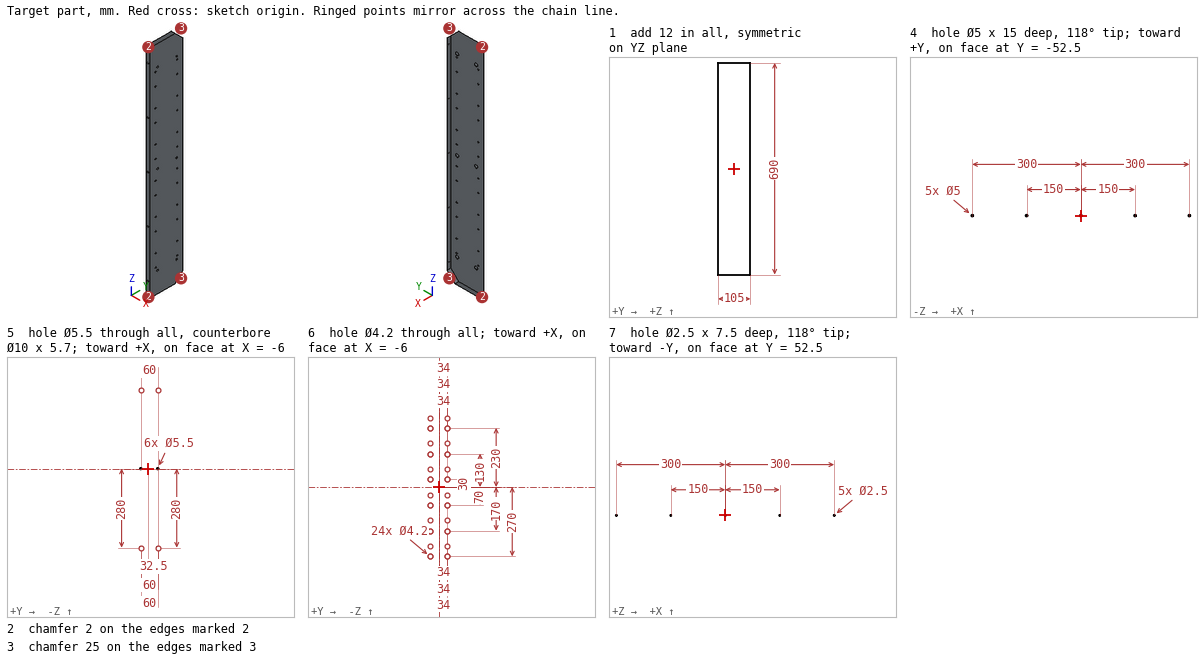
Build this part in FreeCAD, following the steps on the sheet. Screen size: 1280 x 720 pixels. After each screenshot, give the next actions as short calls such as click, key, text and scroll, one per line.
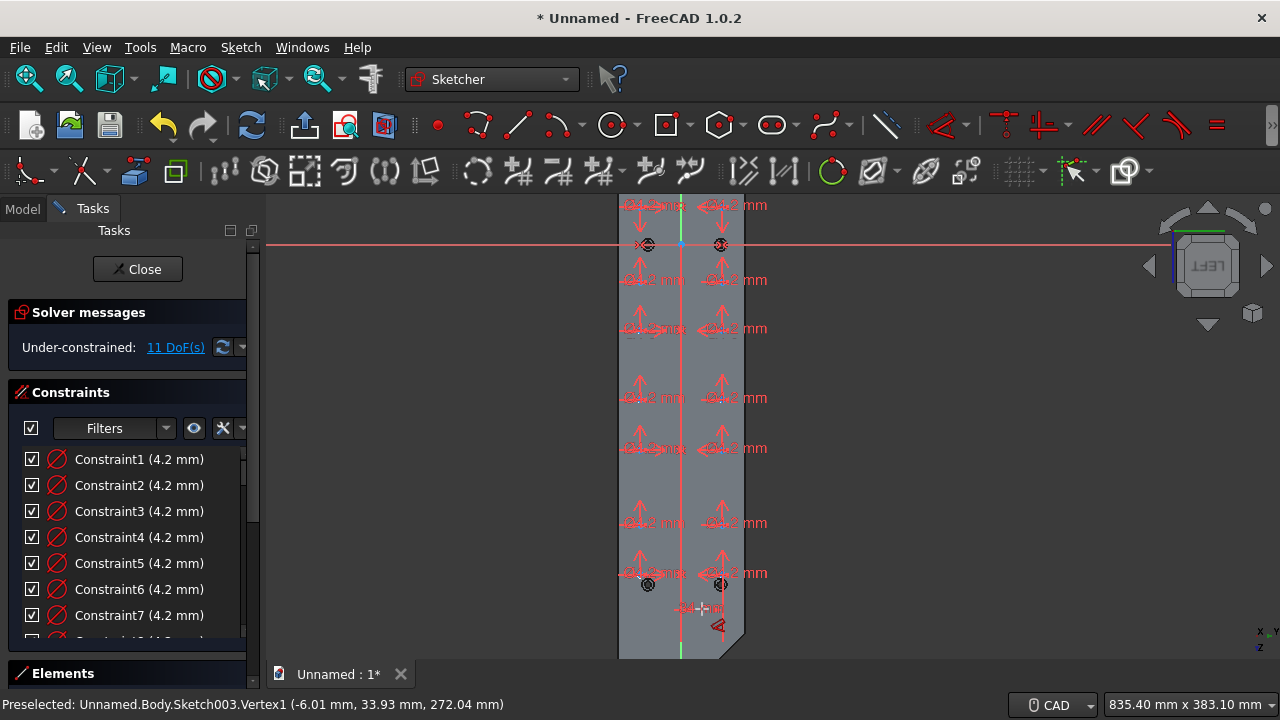
click(722, 450)
click(702, 484)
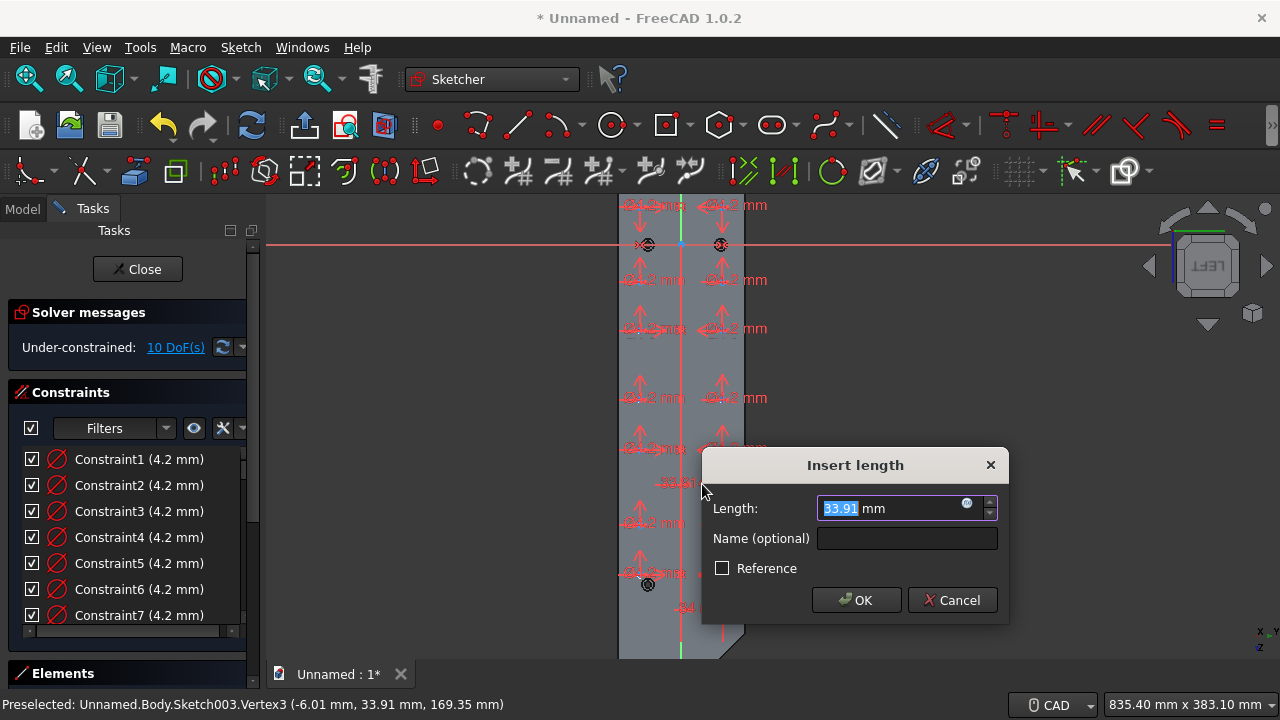
text(34)
key(Return)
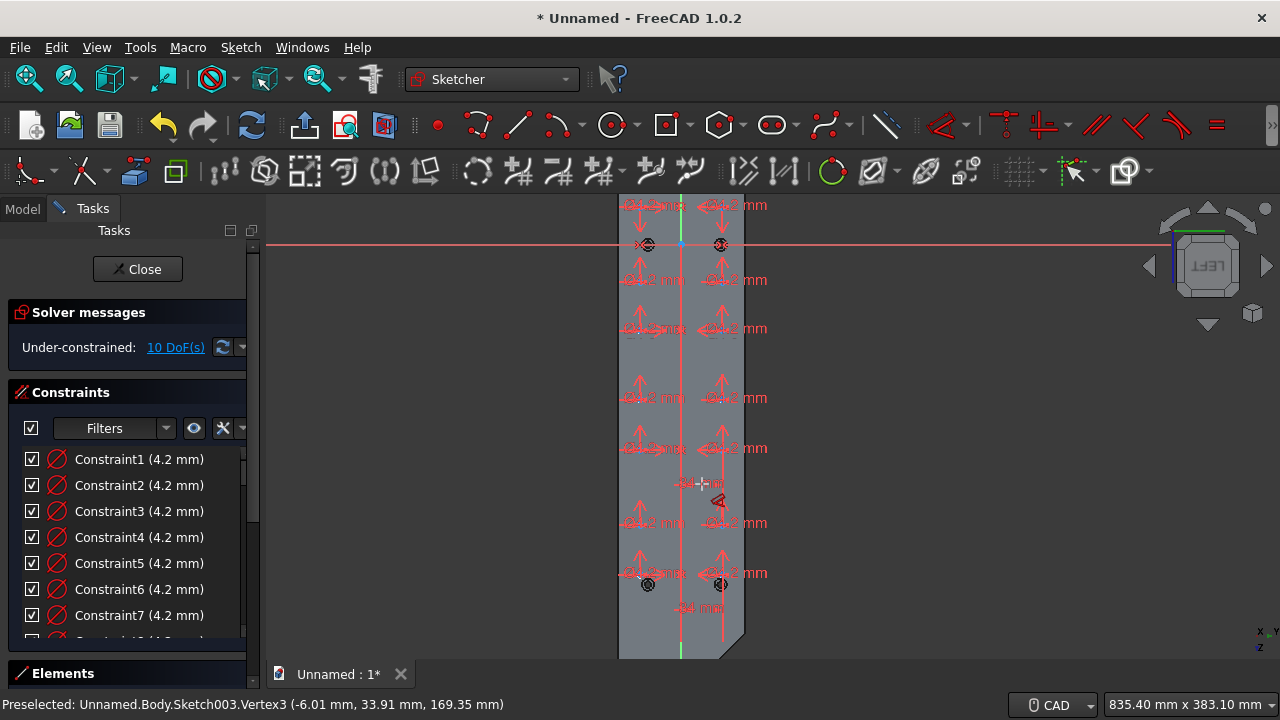
click(722, 331)
click(702, 365)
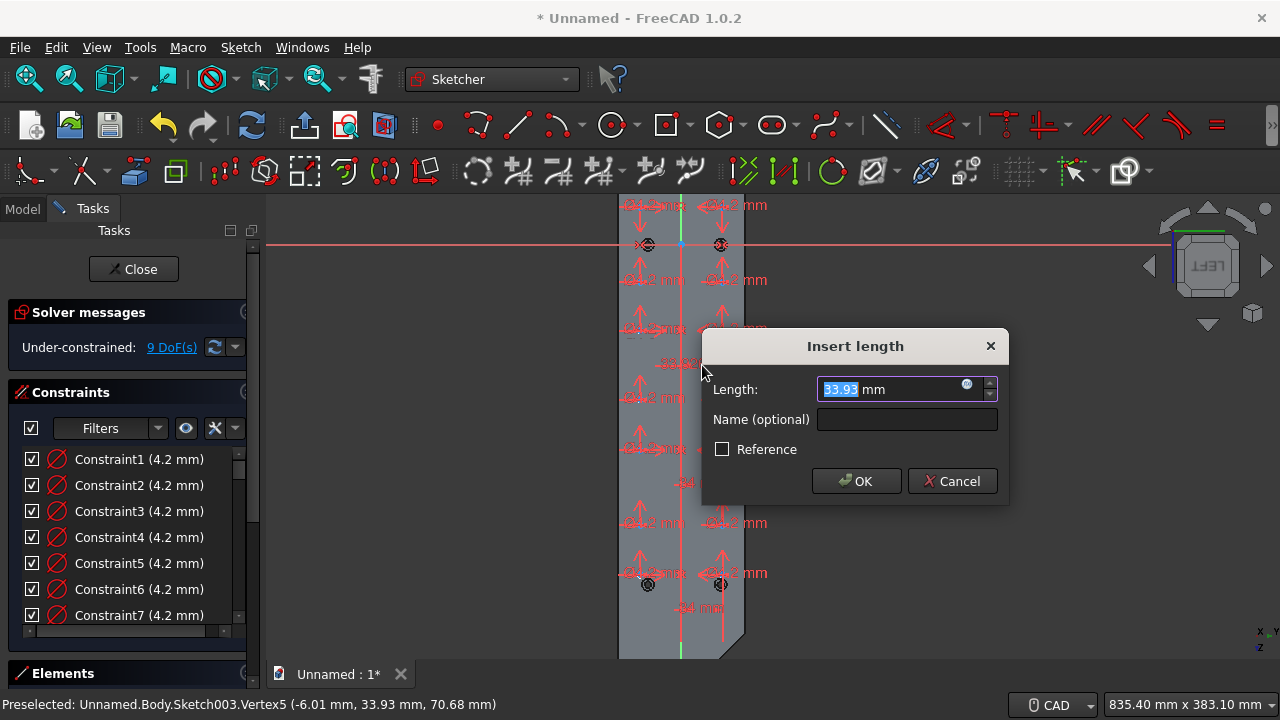
text(34)
key(Return)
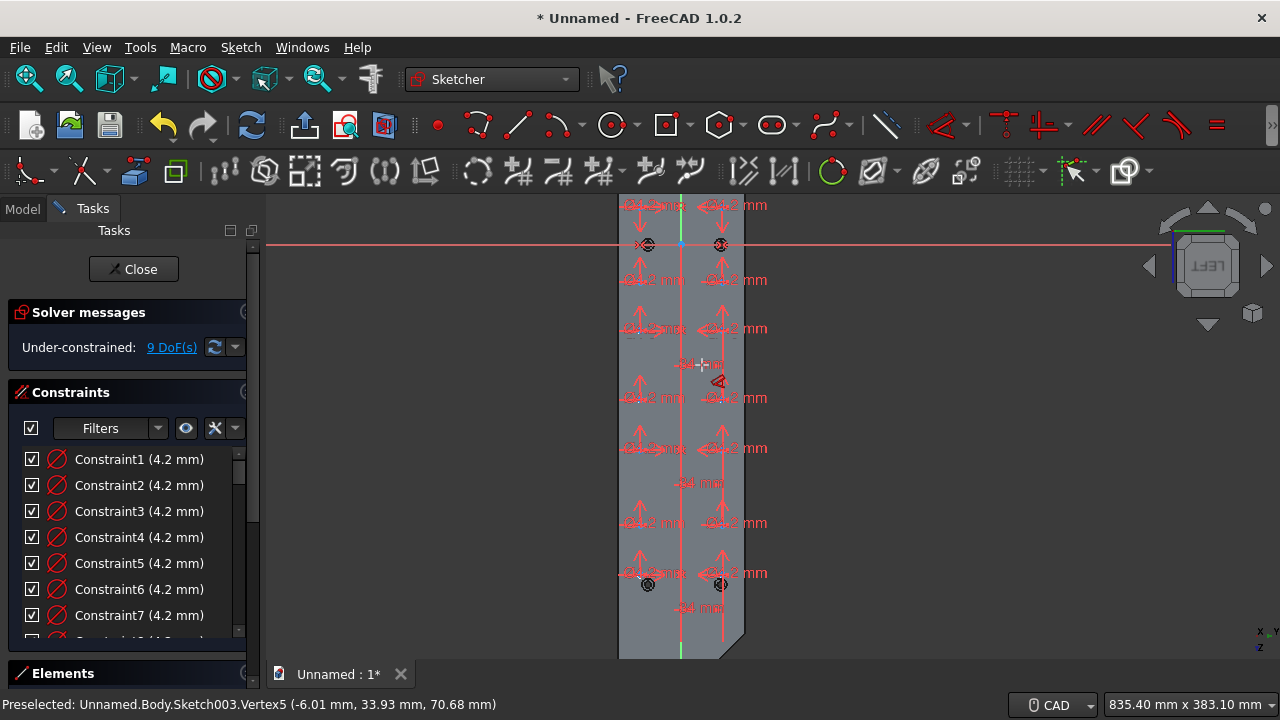
click(723, 331)
click(757, 288)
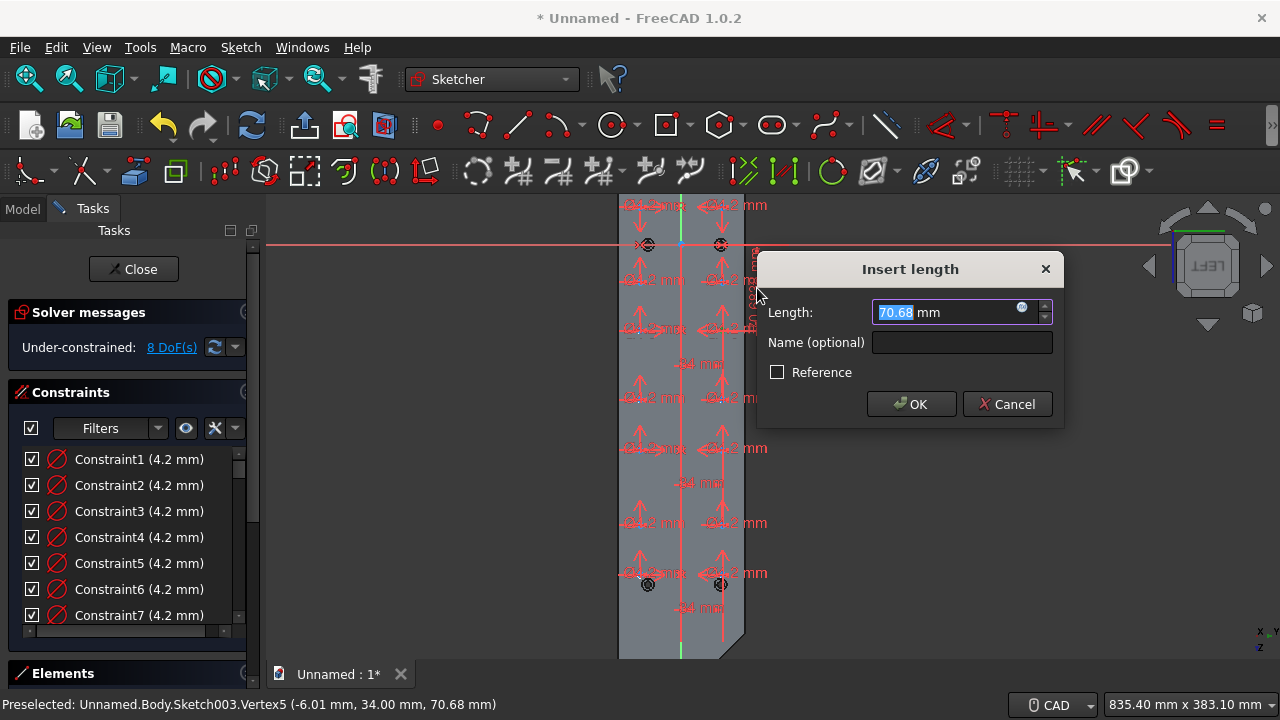
text(70)
key(Return)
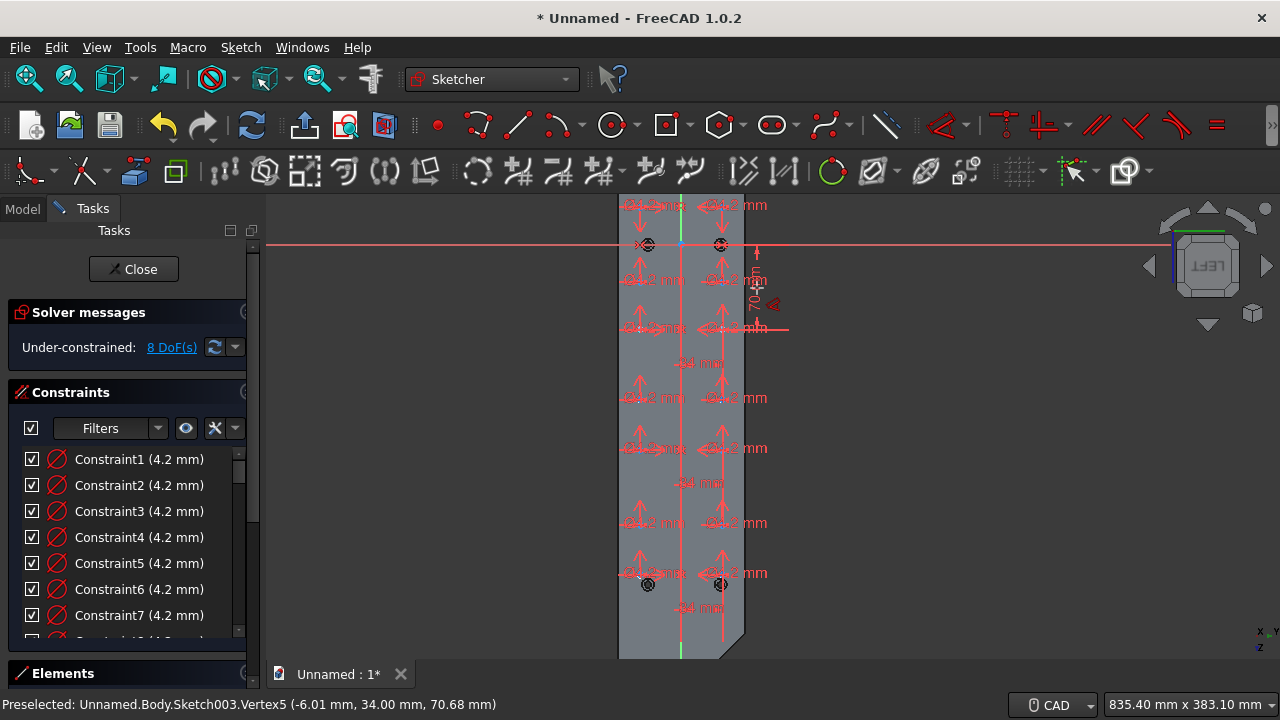
scroll(723, 575, down, 4)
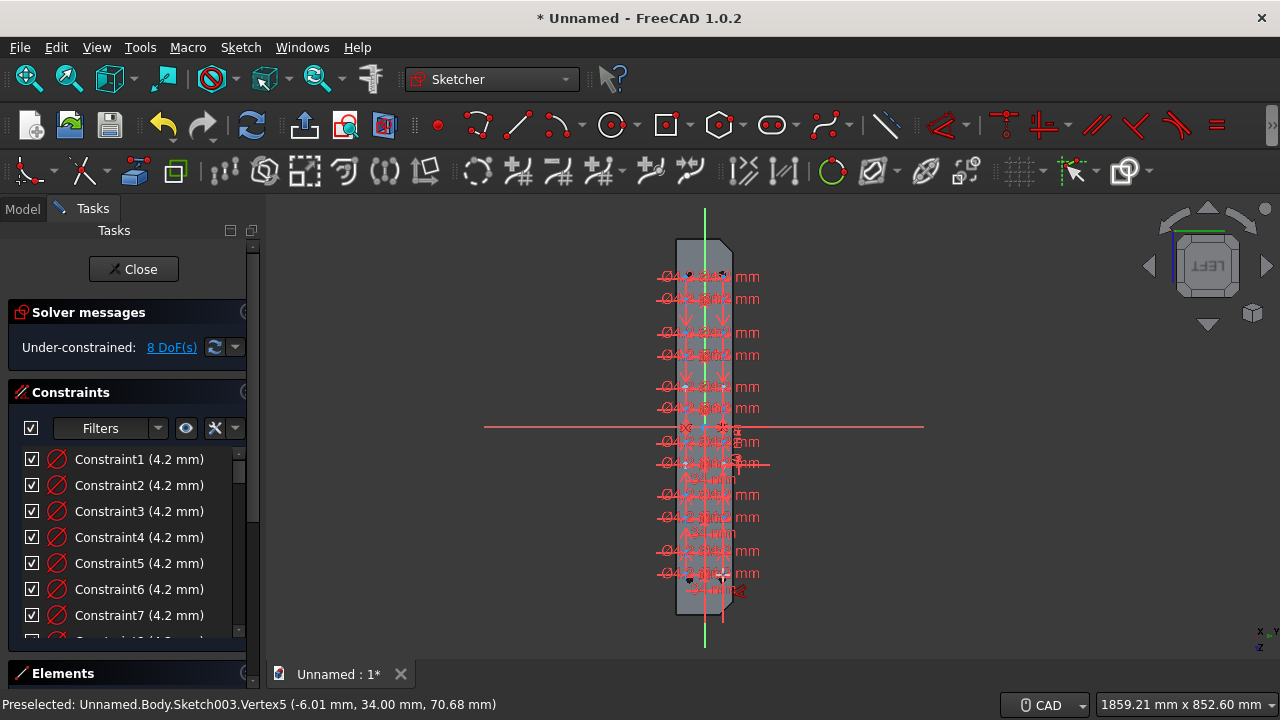
scroll(723, 410, up, 4)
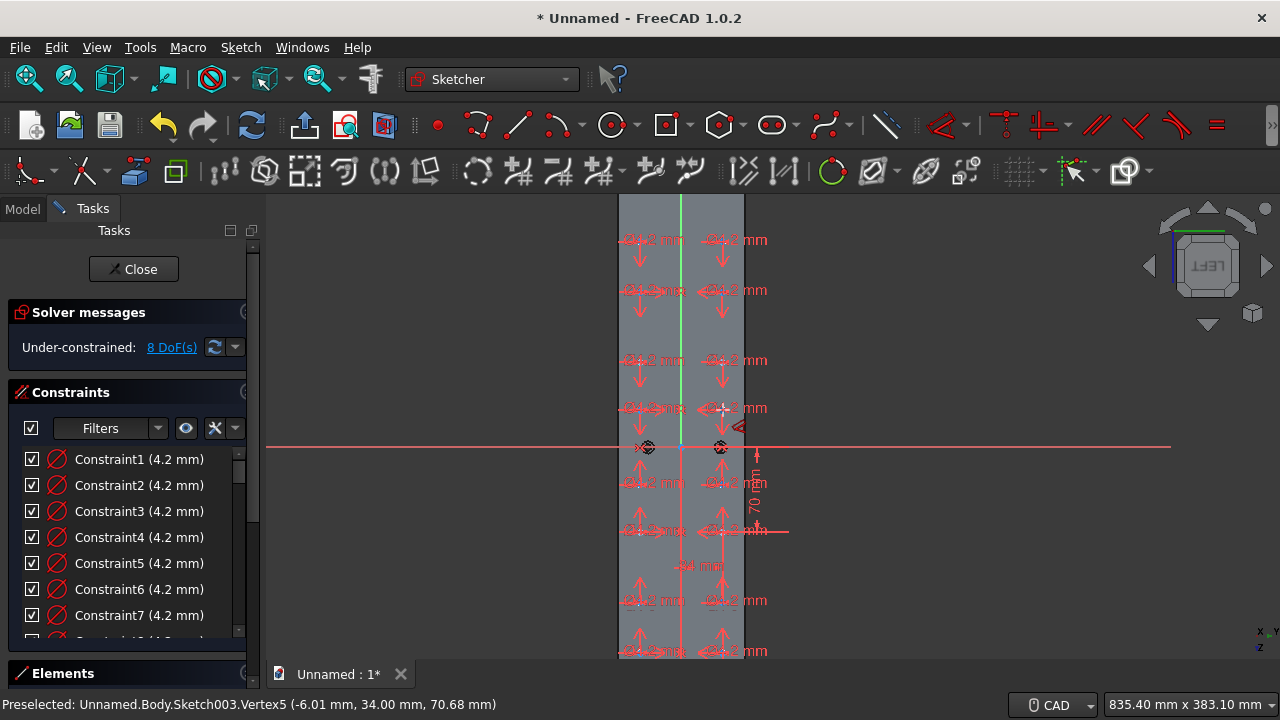
click(722, 410)
click(702, 376)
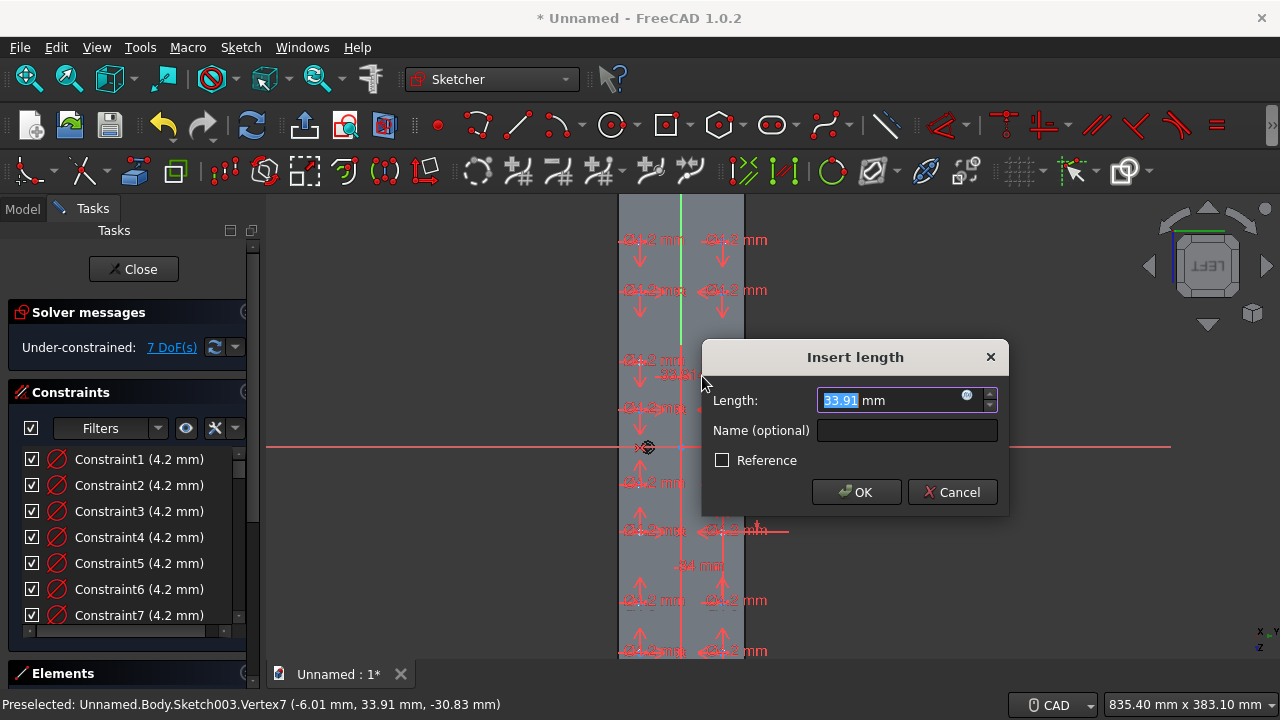
text(34)
key(Return)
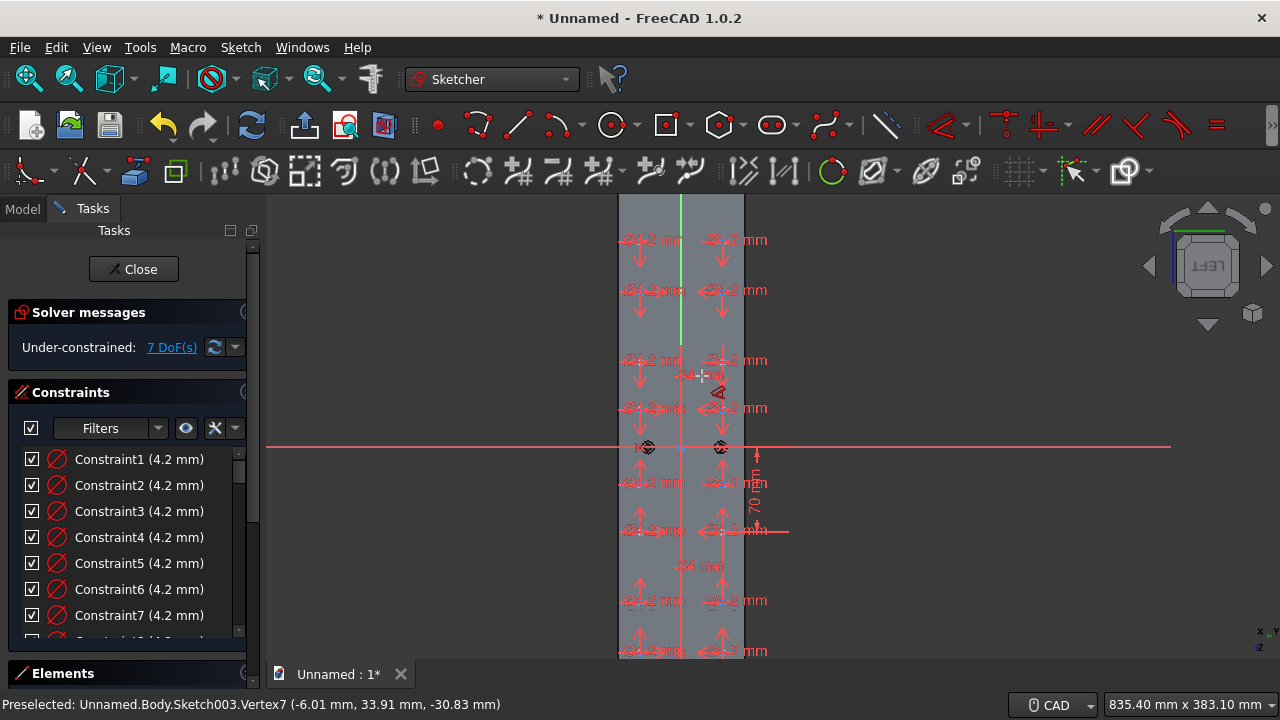
click(723, 410)
click(757, 429)